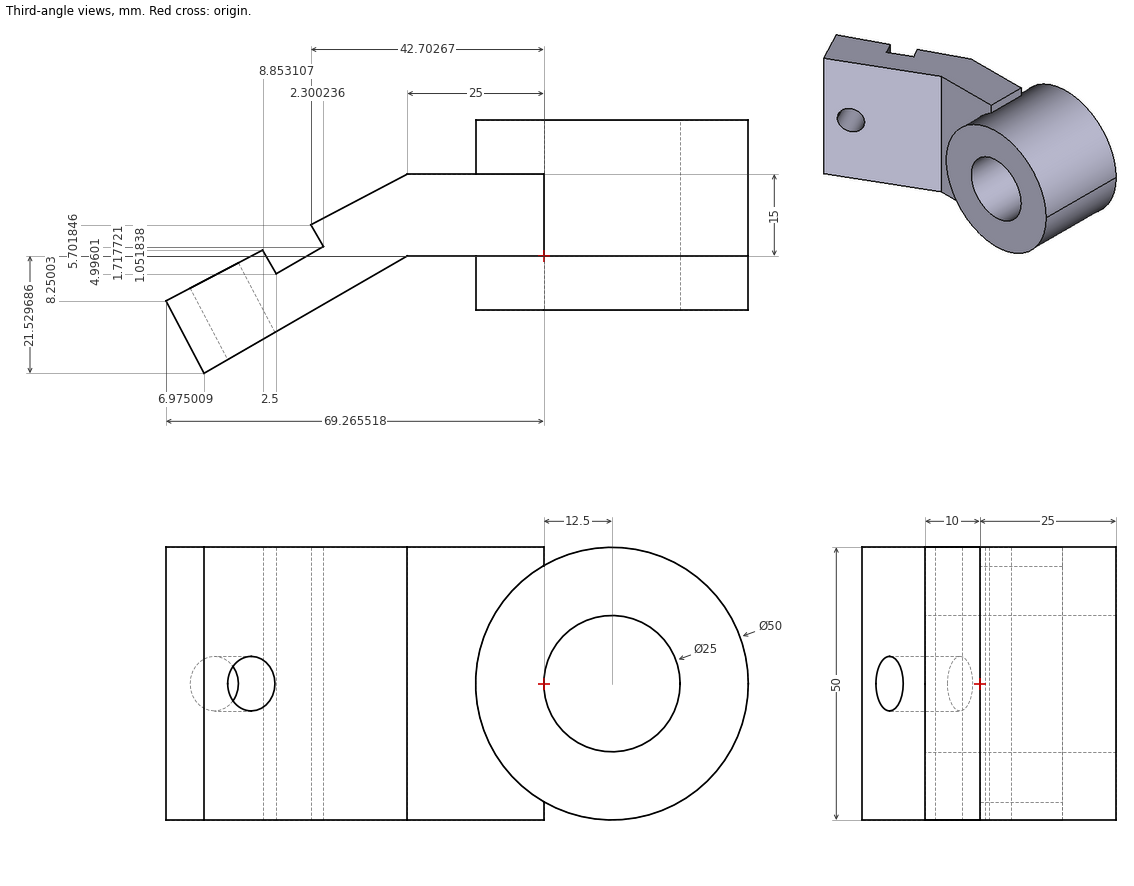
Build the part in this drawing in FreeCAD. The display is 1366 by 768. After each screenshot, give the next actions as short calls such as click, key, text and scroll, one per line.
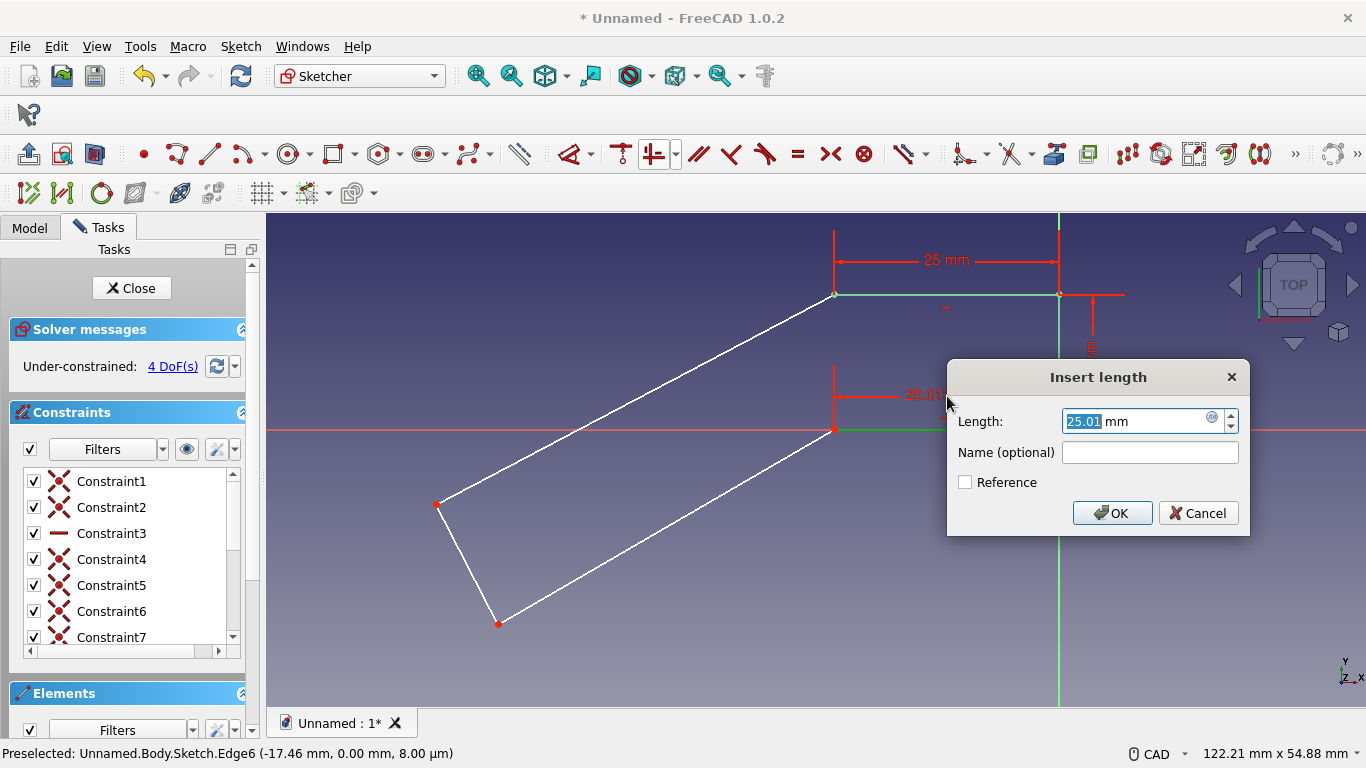
text(25)
key(Return)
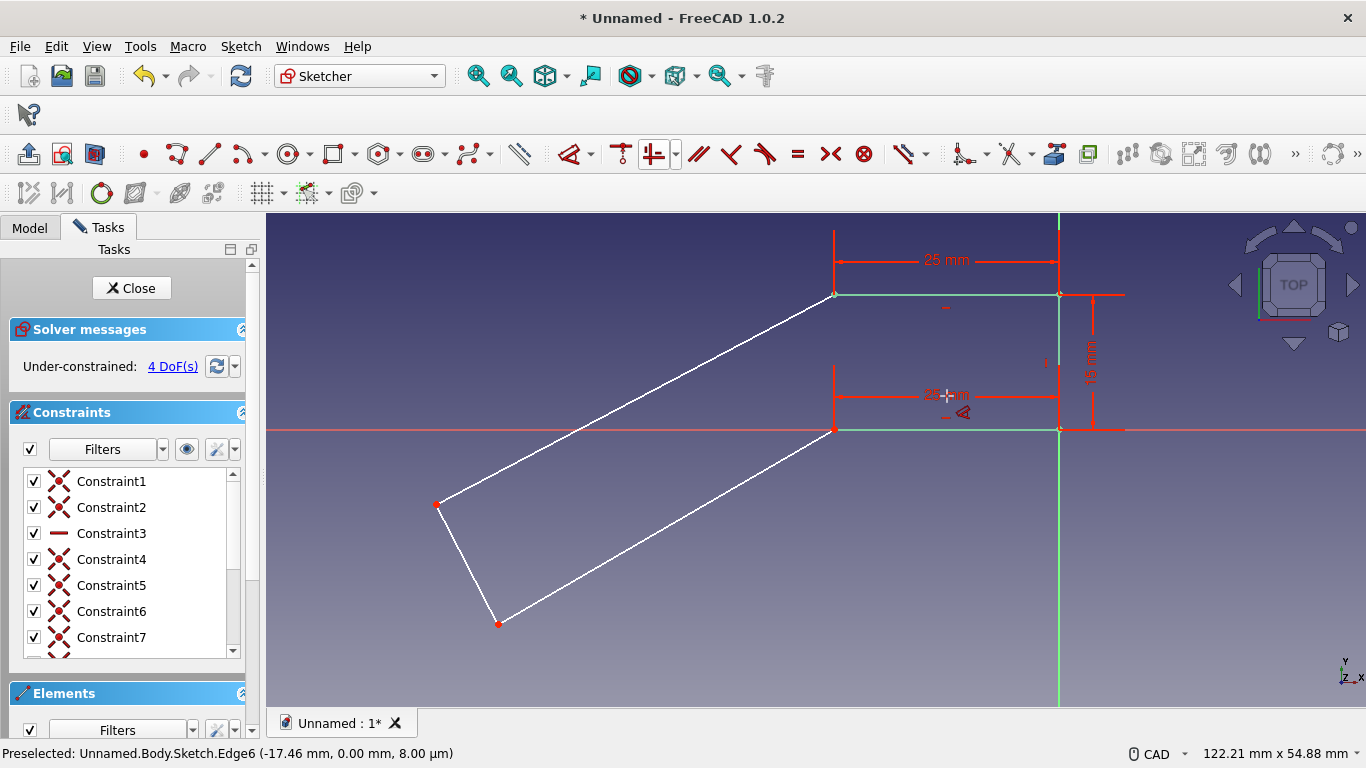
click(436, 505)
click(1093, 467)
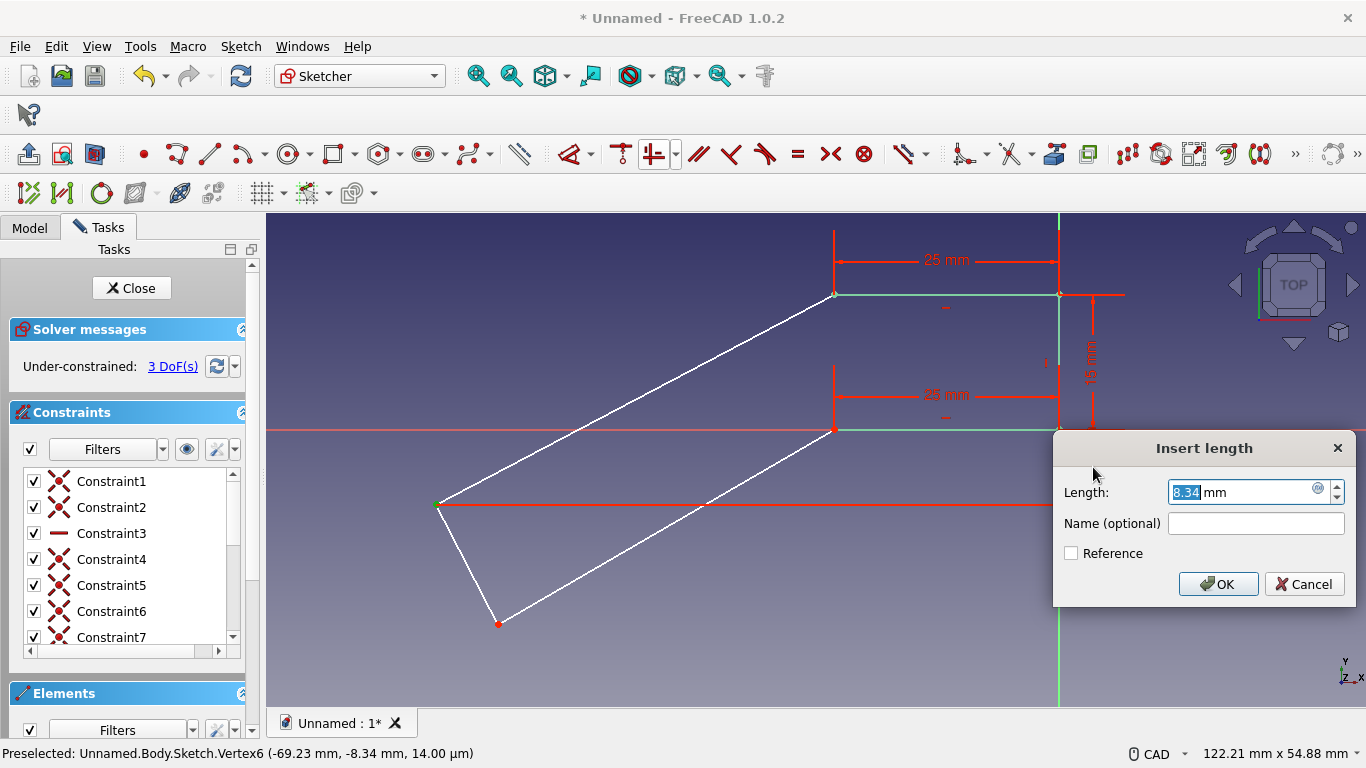
text(8.25003)
key(Return)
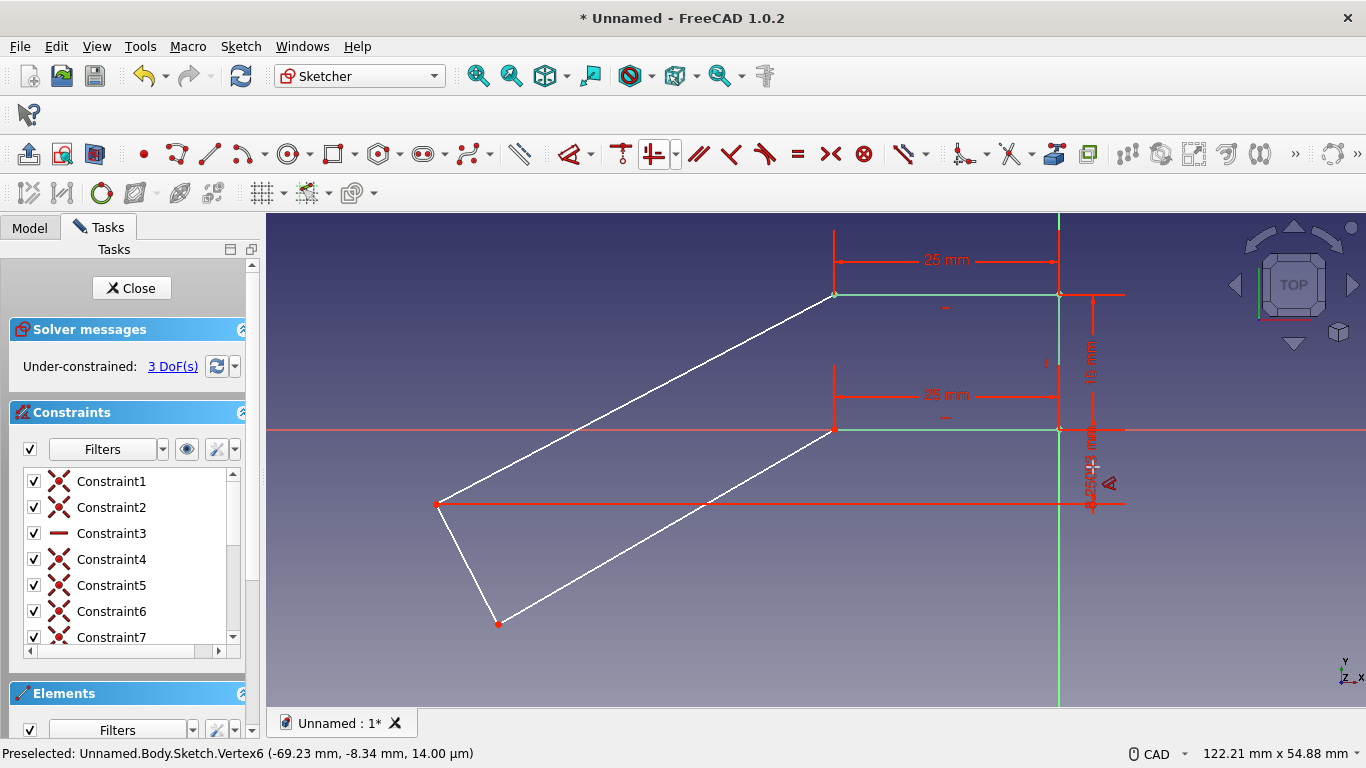
click(455, 540)
click(467, 659)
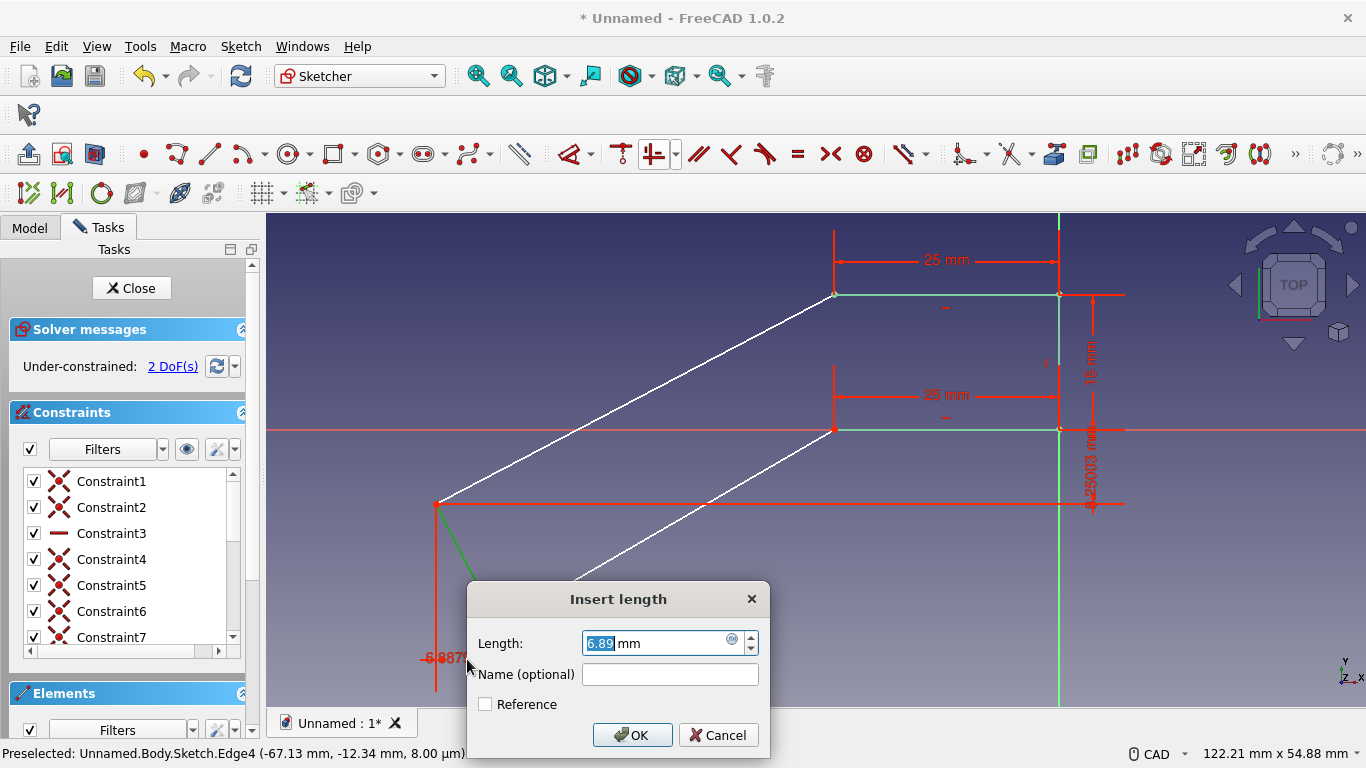
text(6.975009)
key(Return)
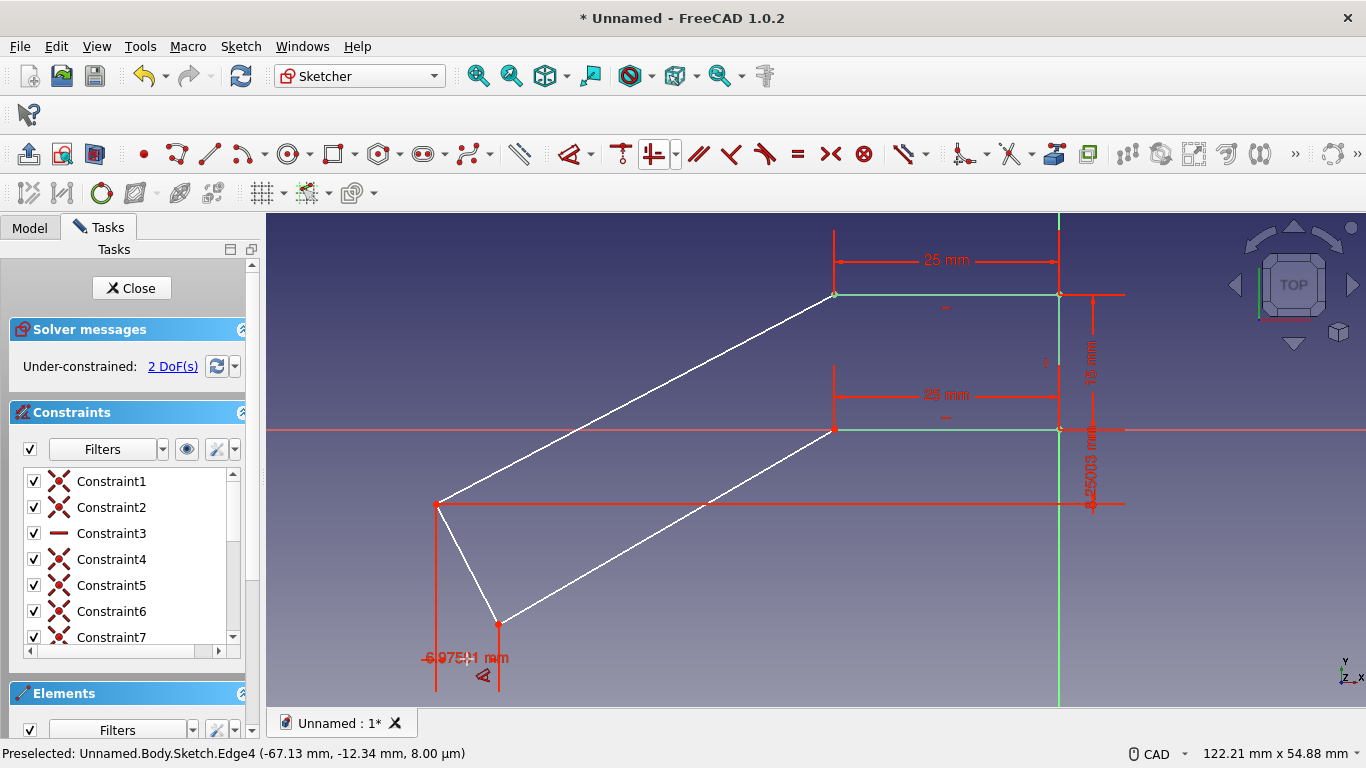
click(436, 504)
click(748, 538)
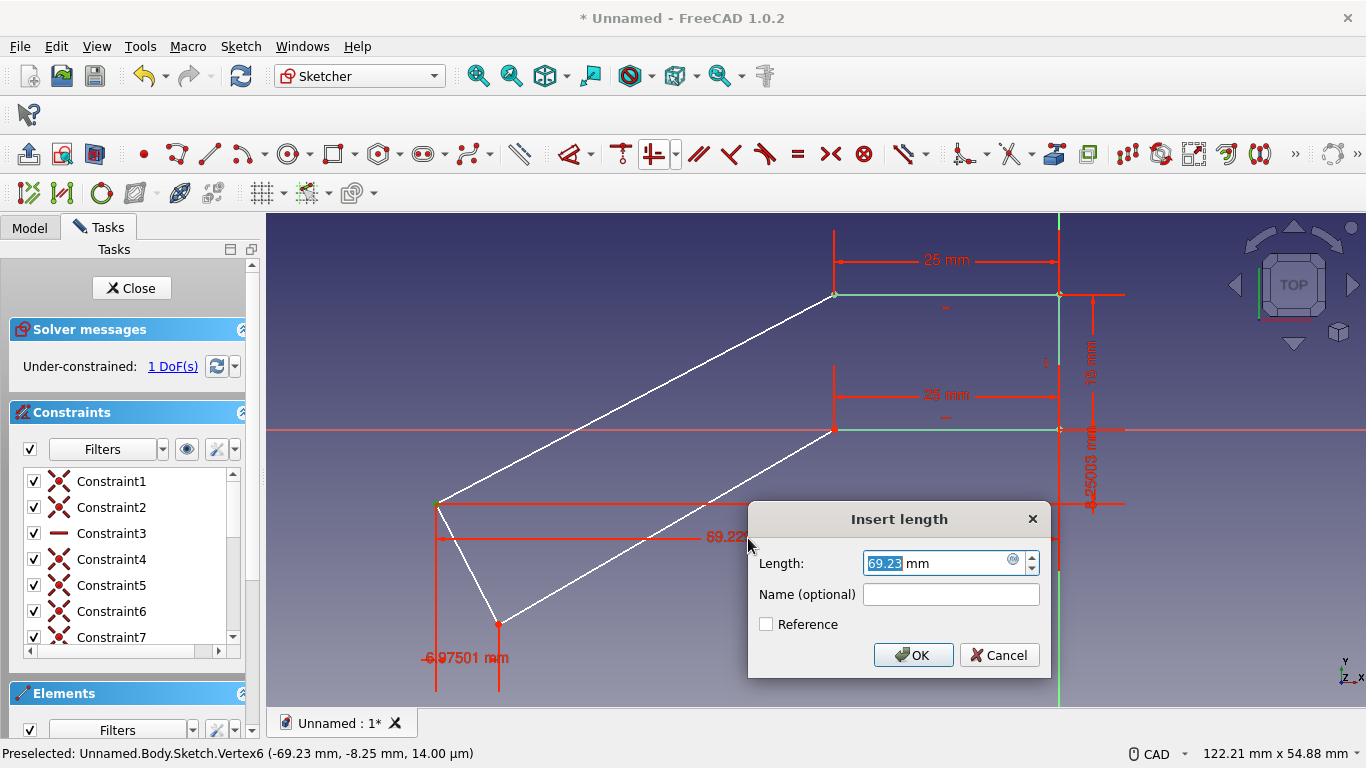
text(69.265518)
key(Return)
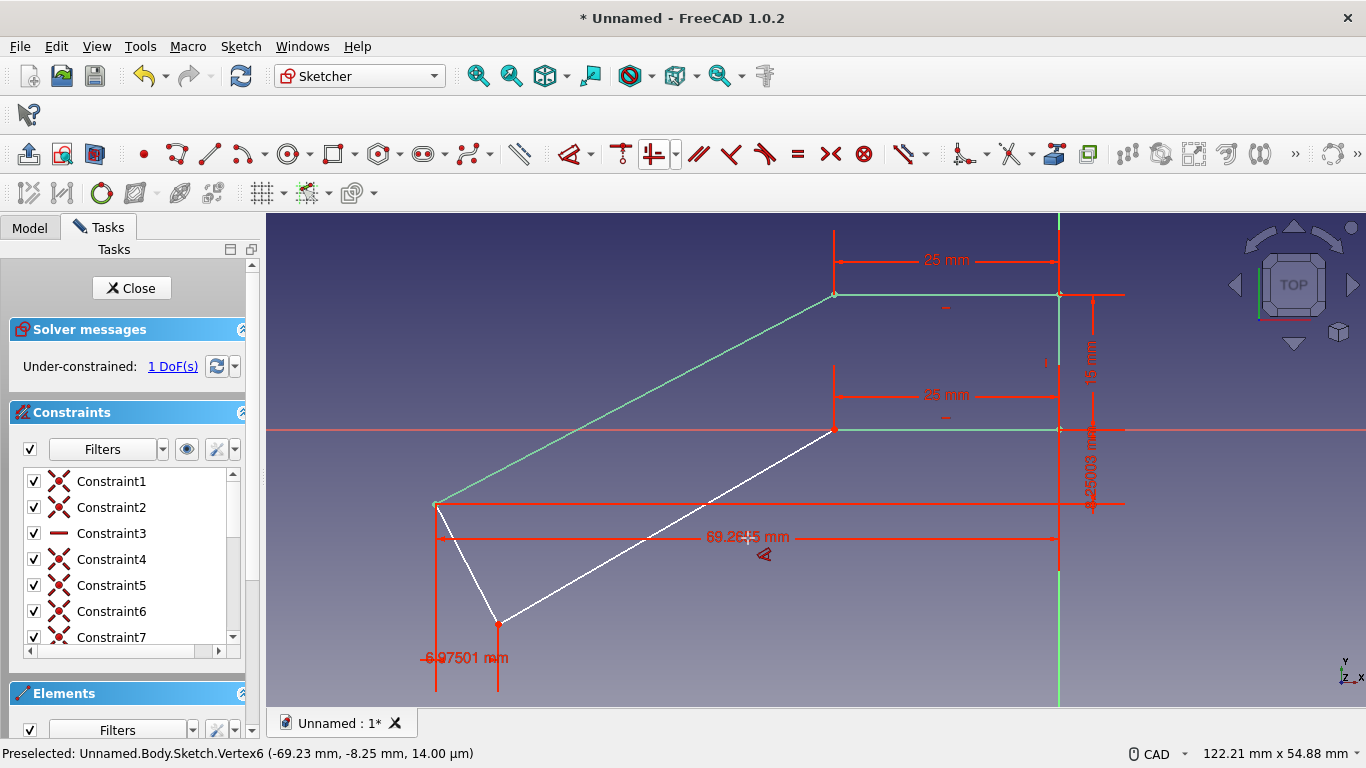
click(498, 625)
click(1093, 527)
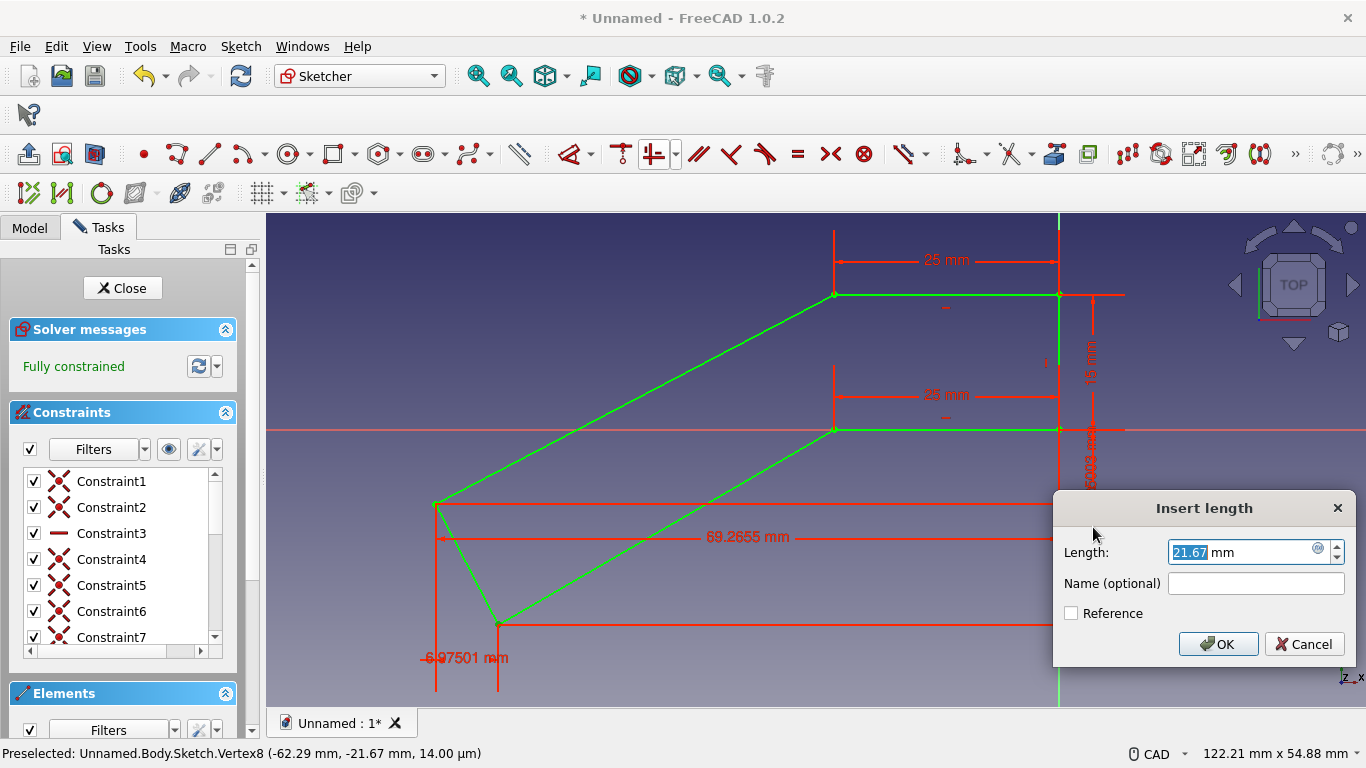
text(21.529686)
key(Return)
key(Escape)